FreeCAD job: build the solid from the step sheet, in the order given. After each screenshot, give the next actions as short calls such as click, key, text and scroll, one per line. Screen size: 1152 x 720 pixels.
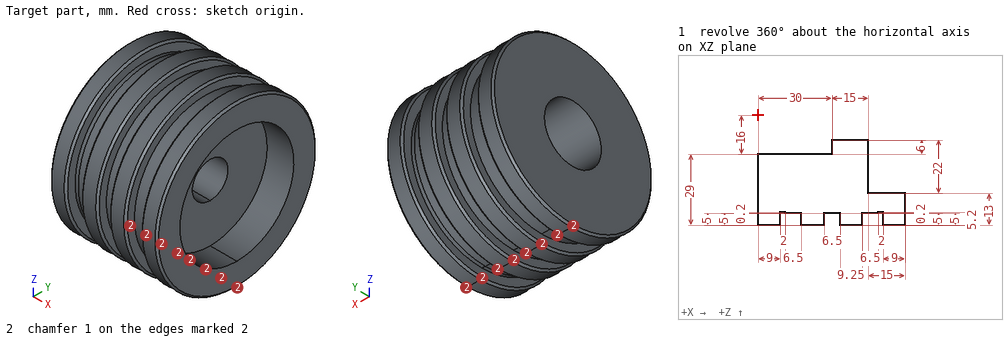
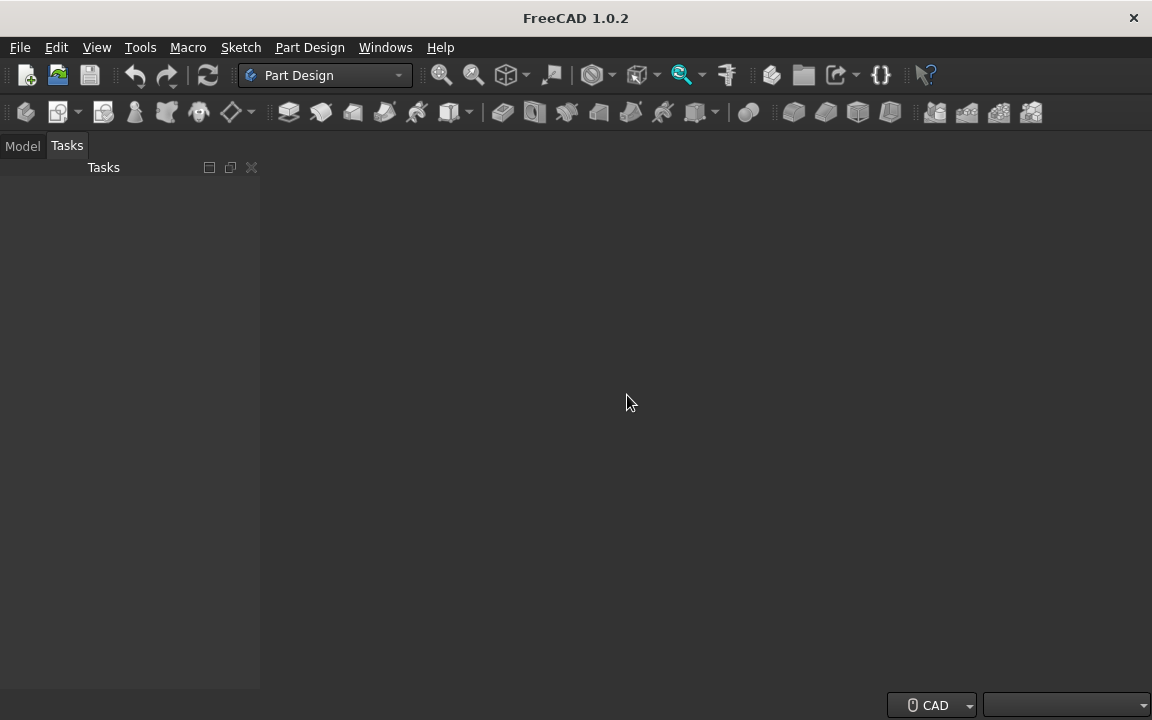
click(26, 76)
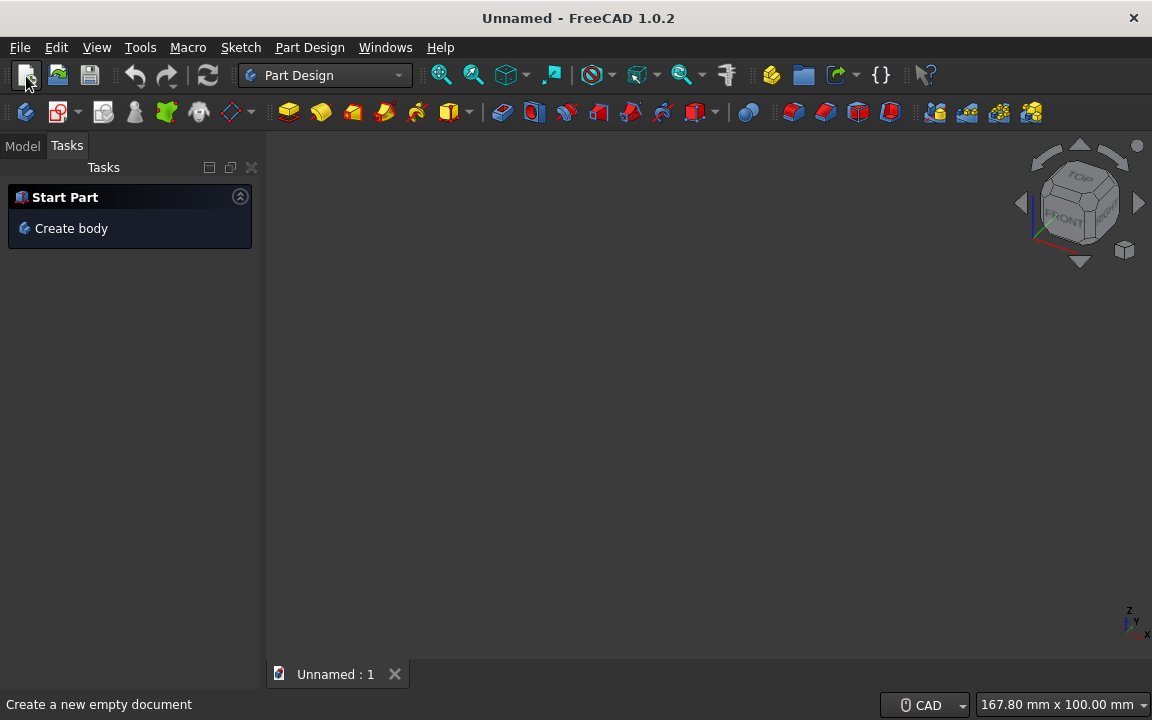
click(58, 112)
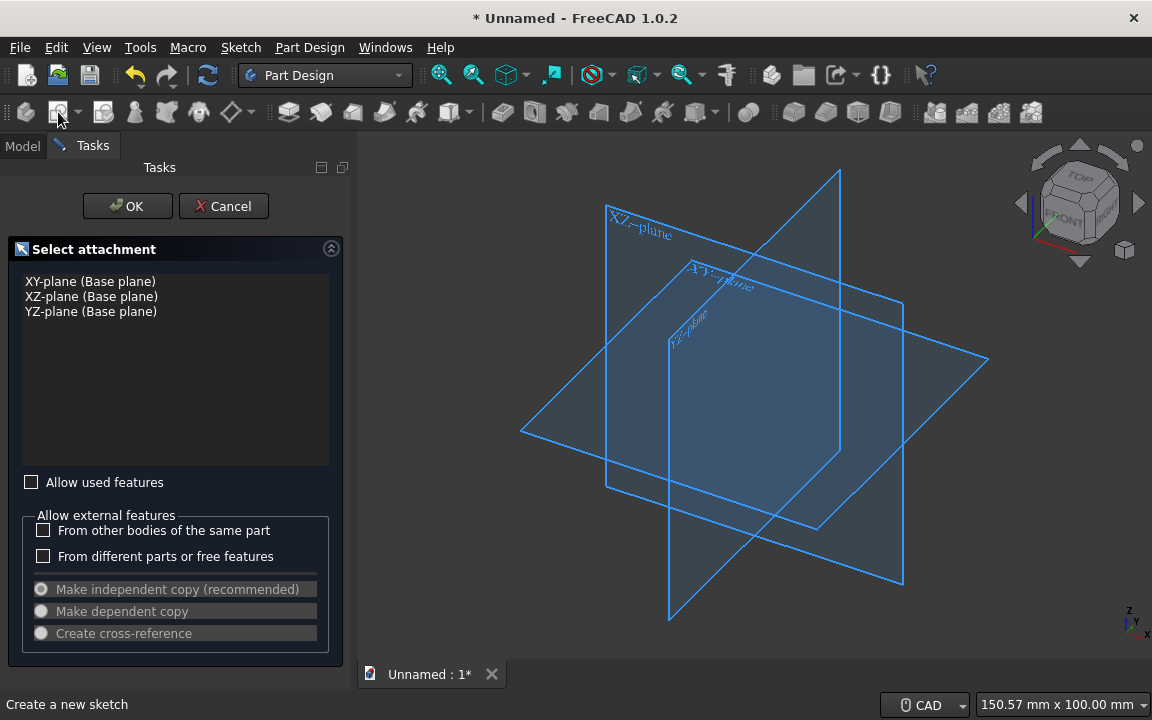
click(82, 296)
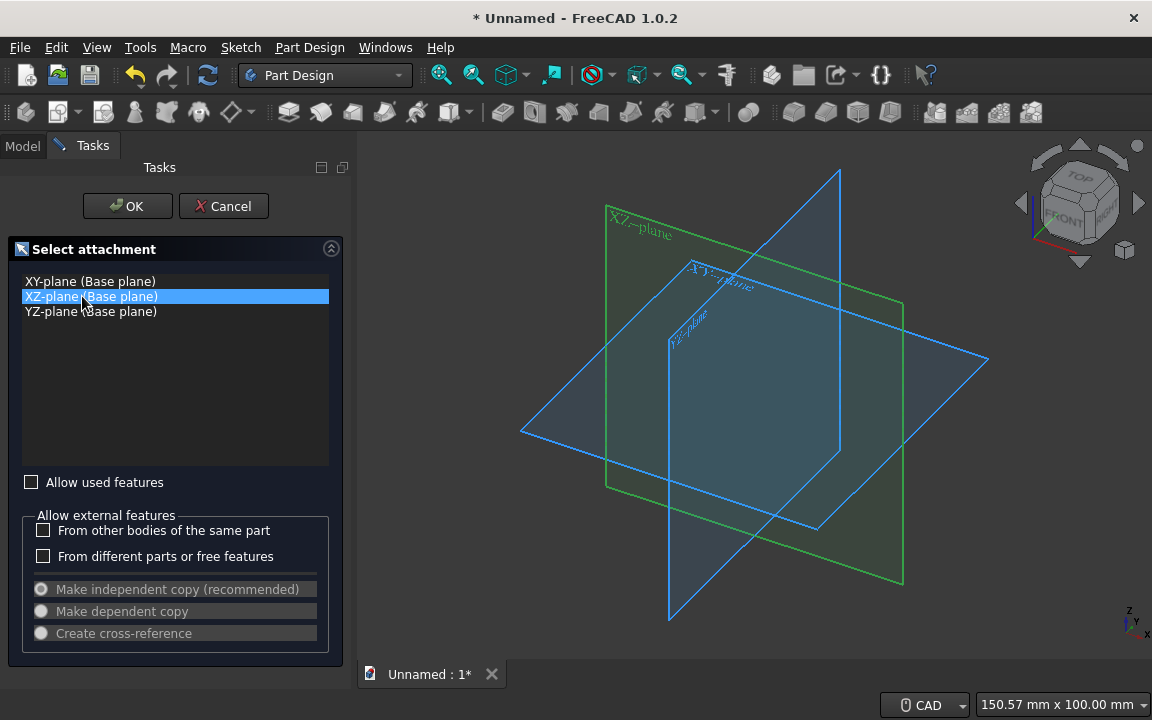
click(128, 206)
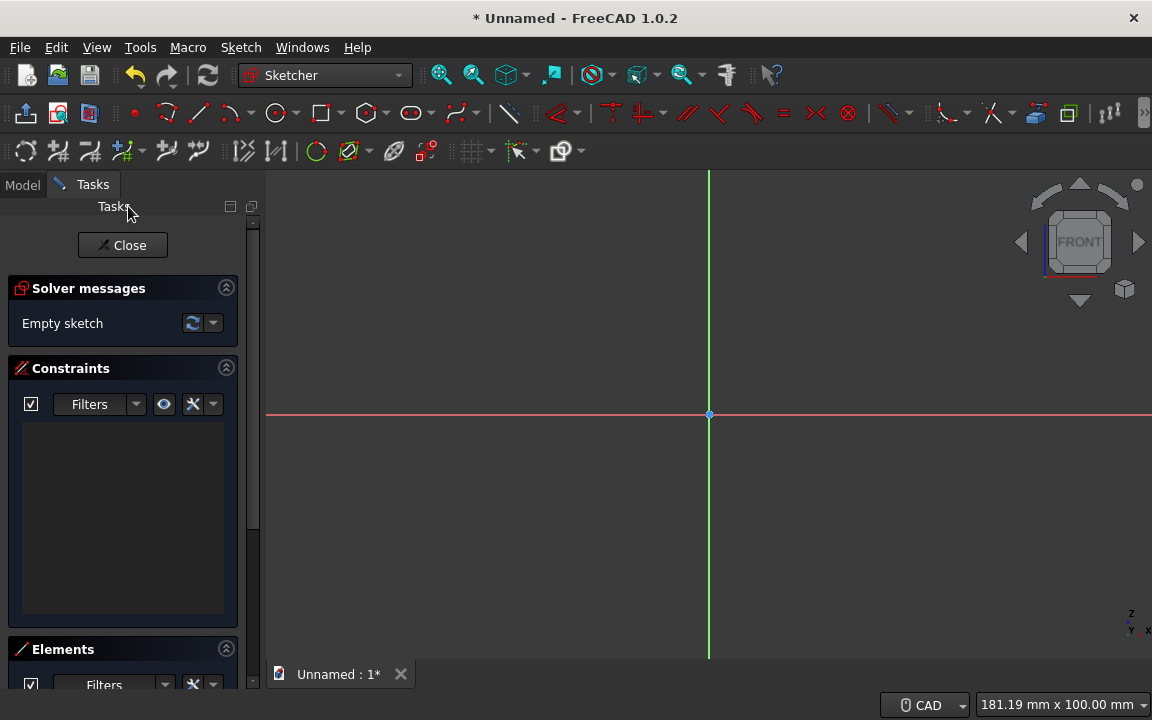
scroll(294, 198, down, 1)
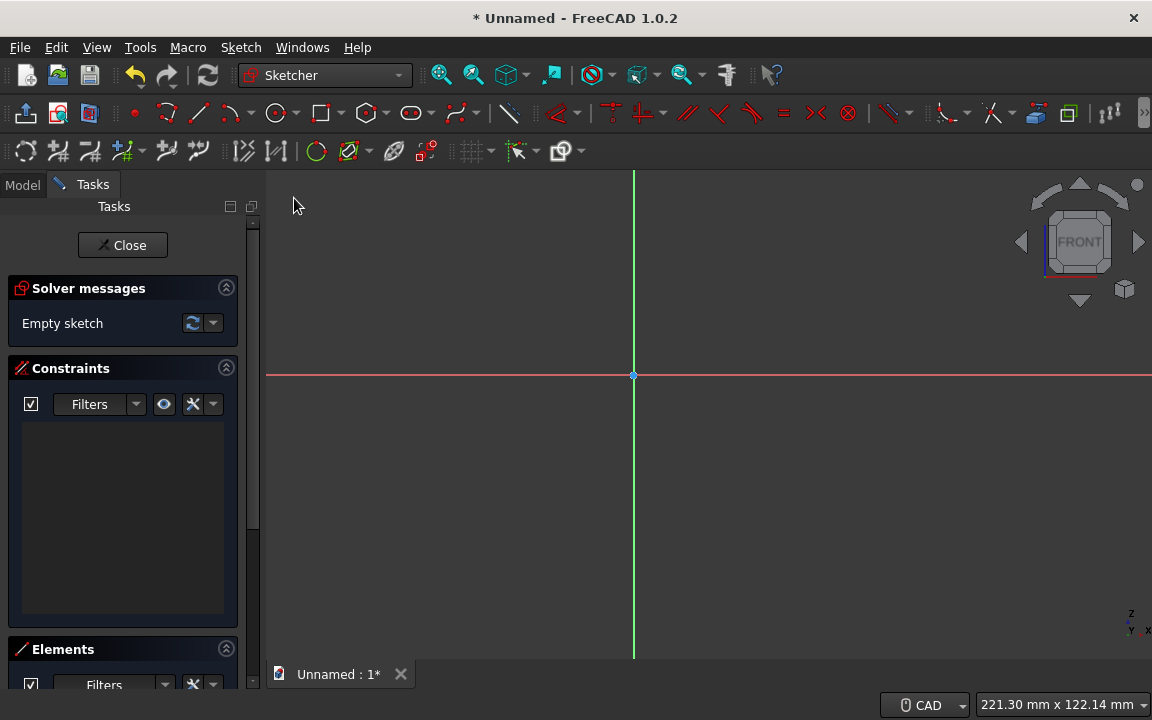
scroll(892, 527, up, 3)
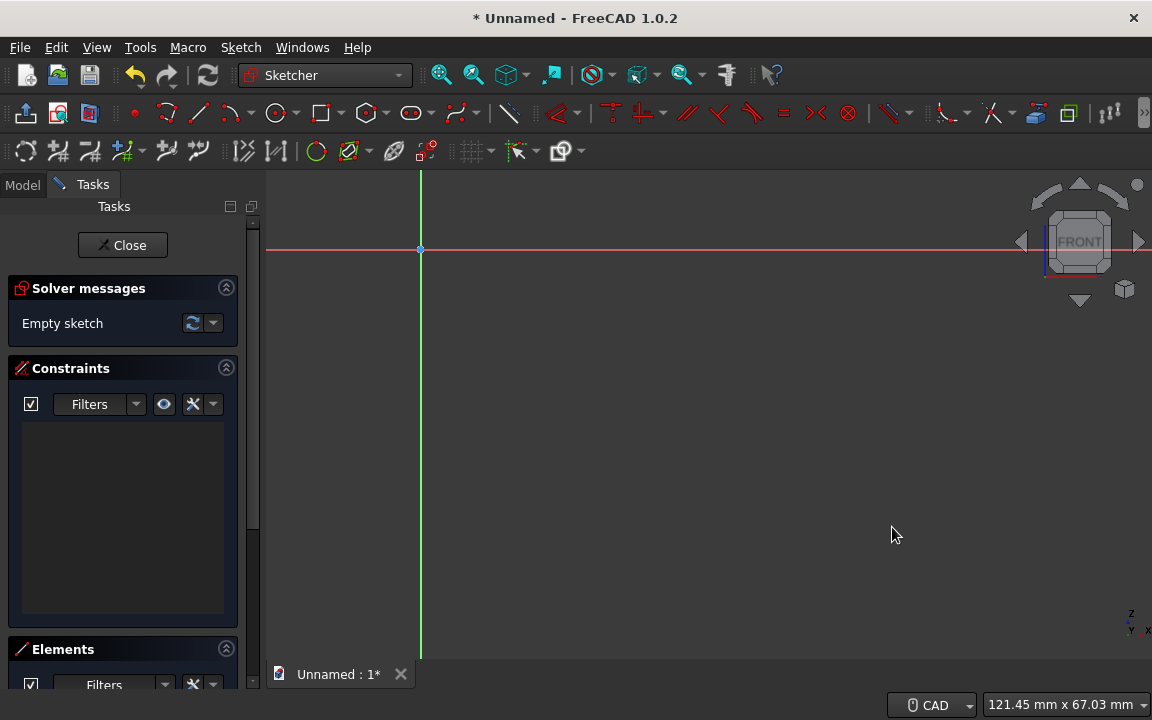
click(168, 114)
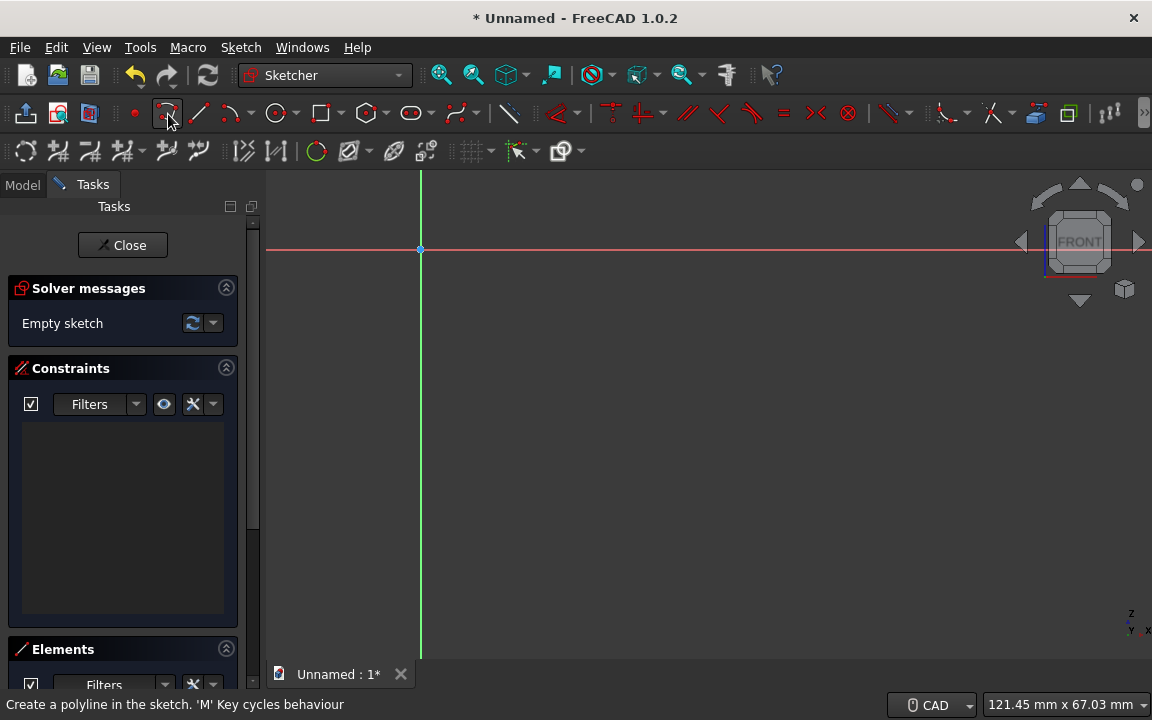
click(421, 367)
click(640, 367)
click(640, 323)
click(749, 323)
click(749, 483)
click(859, 483)
click(859, 578)
click(793, 578)
click(793, 540)
click(778, 540)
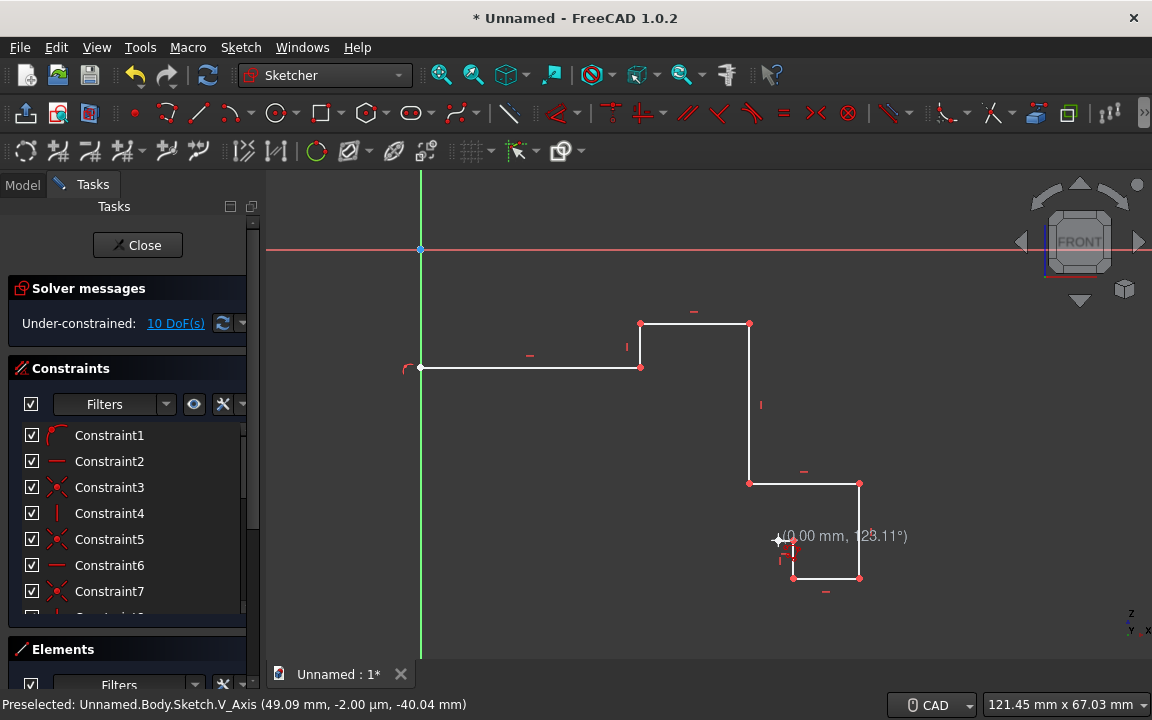
scroll(778, 542, up, 12)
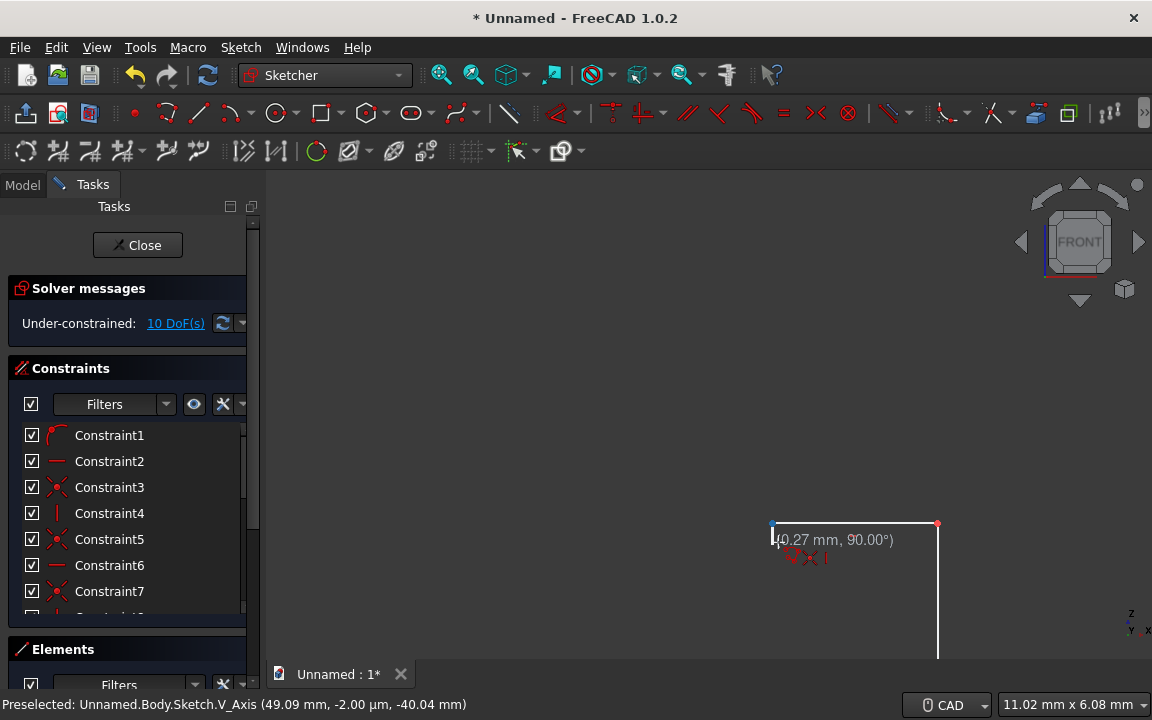
click(772, 531)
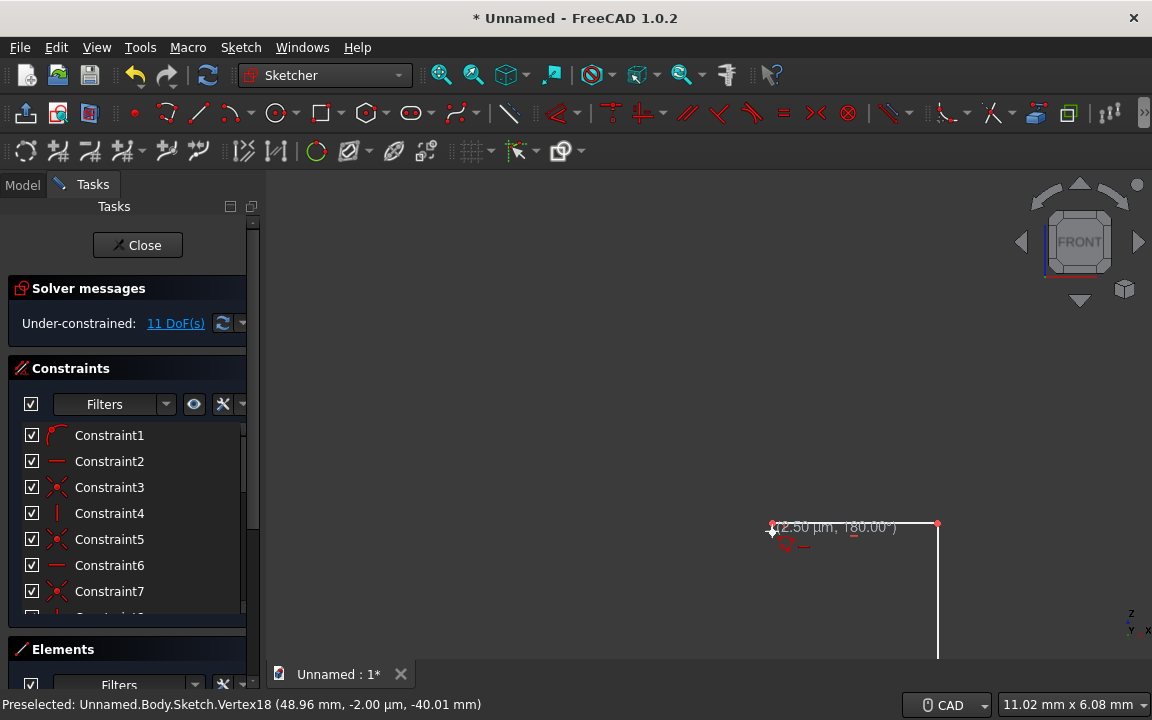
scroll(779, 543, down, 12)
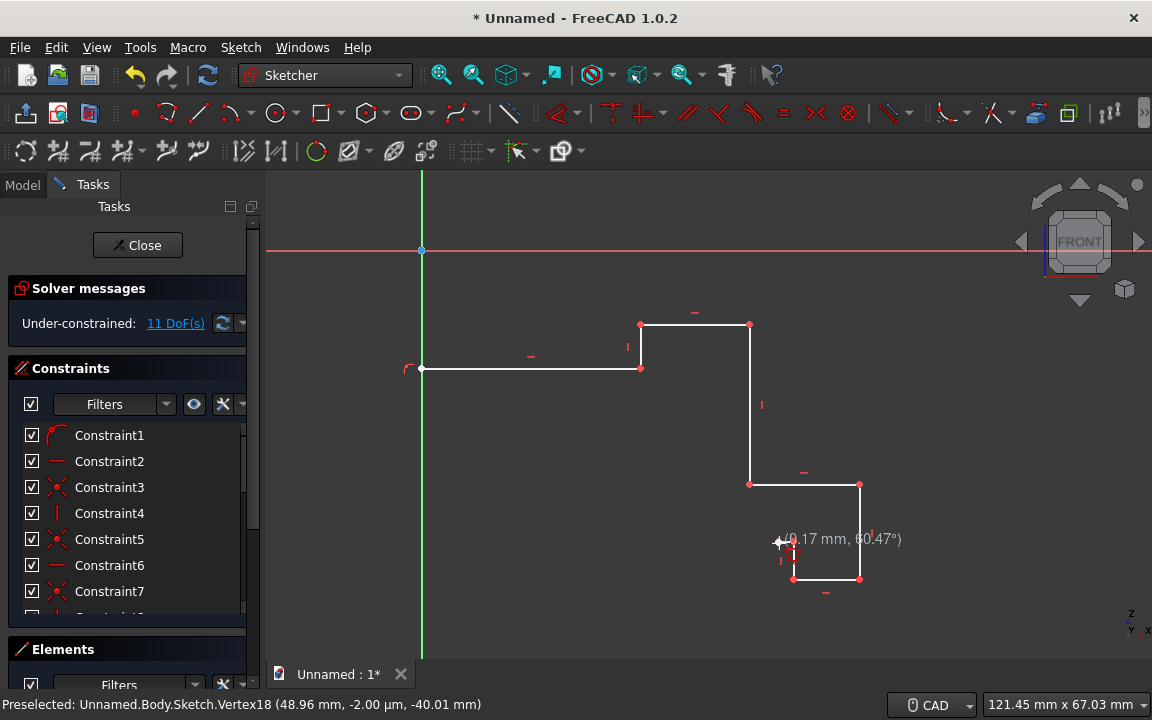
click(732, 543)
click(732, 579)
click(664, 579)
click(664, 543)
click(617, 543)
click(617, 579)
click(549, 579)
click(549, 543)
click(502, 543)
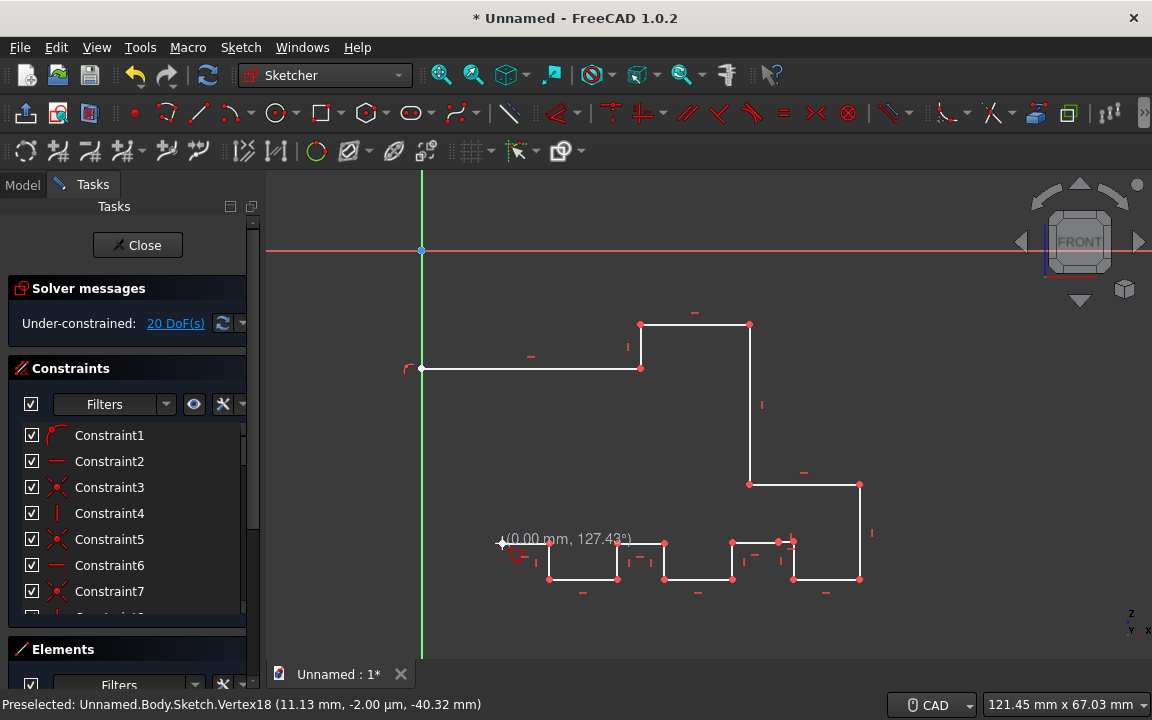
scroll(502, 541, up, 12)